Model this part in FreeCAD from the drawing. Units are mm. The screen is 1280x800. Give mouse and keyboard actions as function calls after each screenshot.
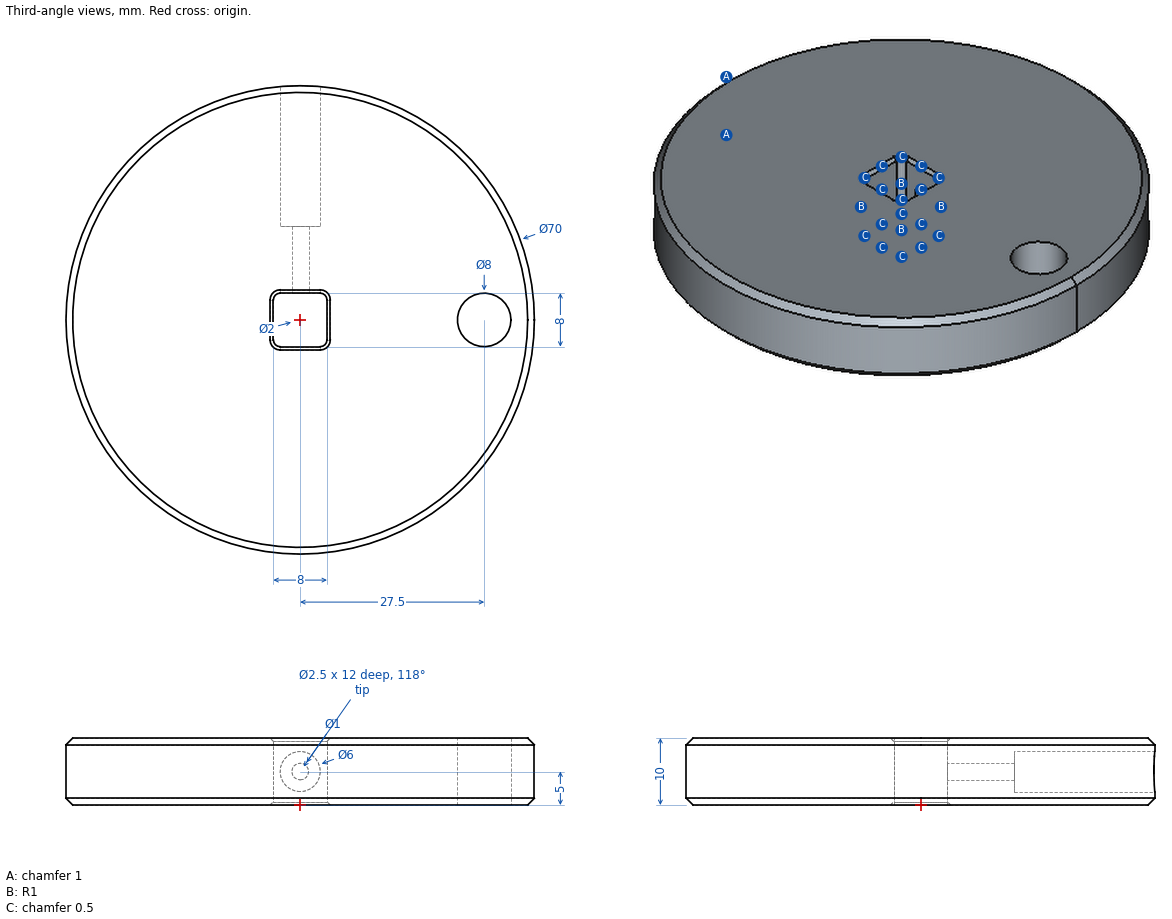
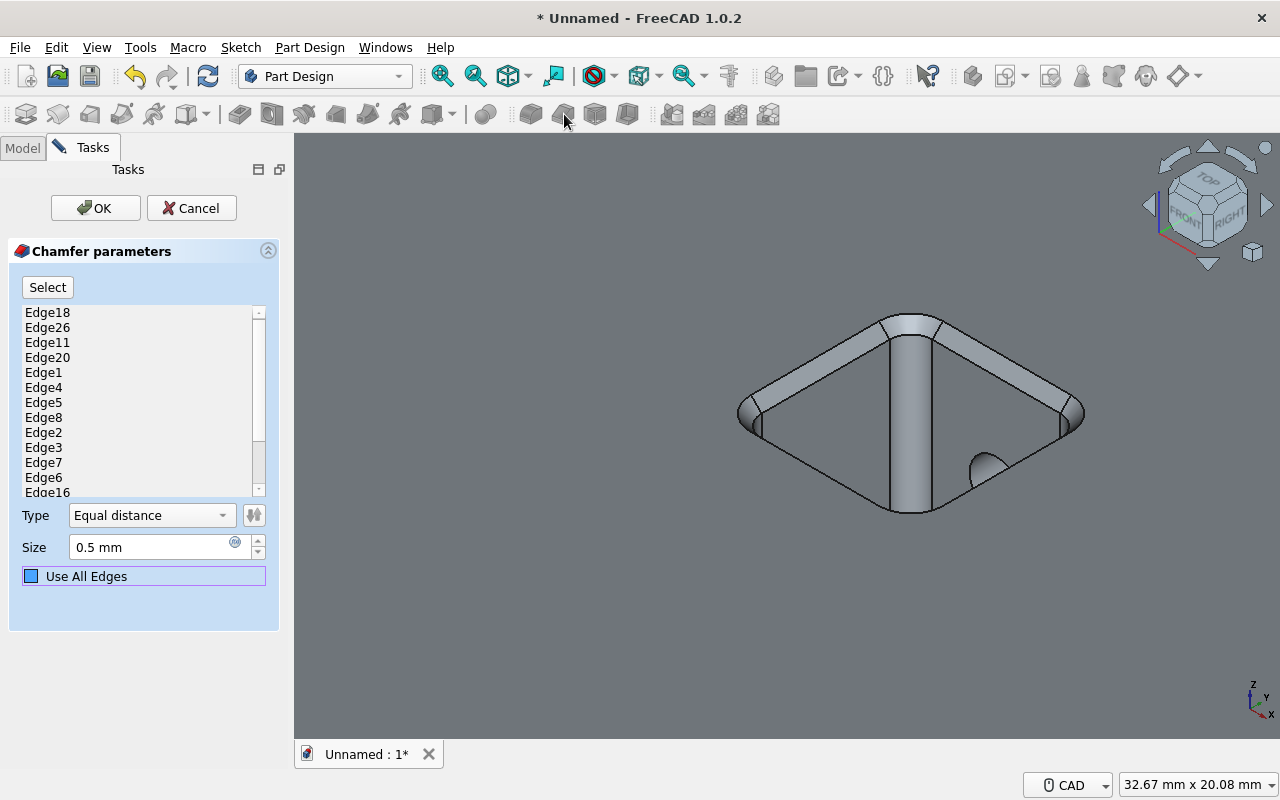
click(96, 208)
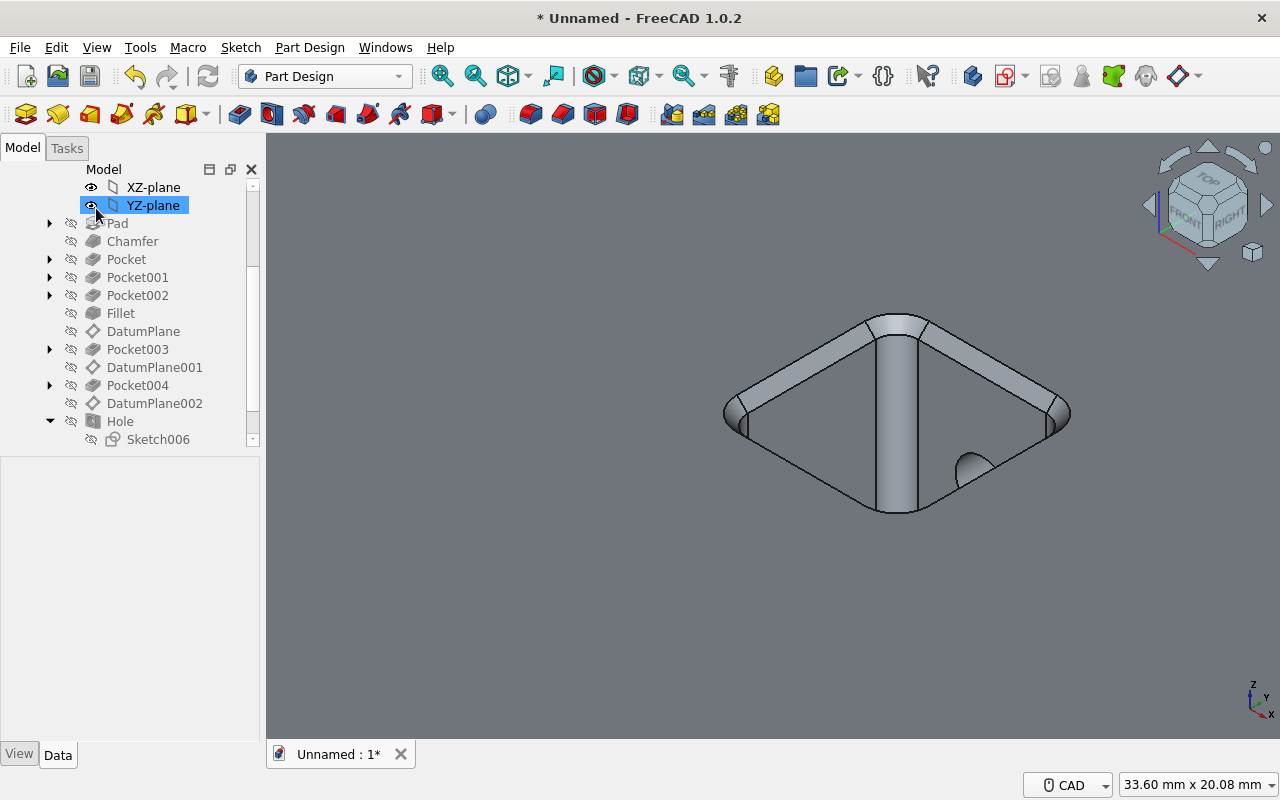
click(444, 76)